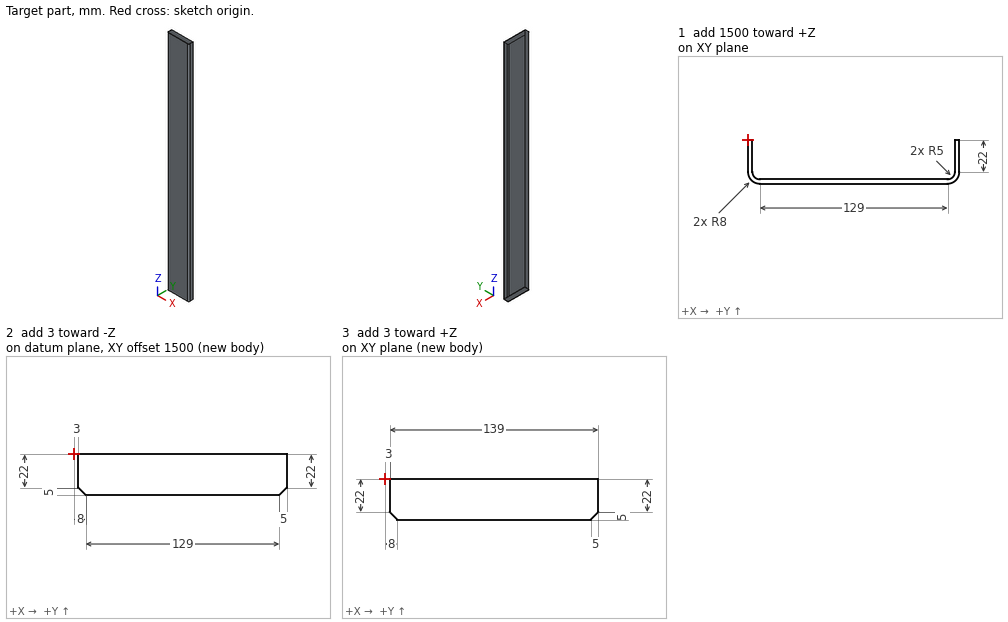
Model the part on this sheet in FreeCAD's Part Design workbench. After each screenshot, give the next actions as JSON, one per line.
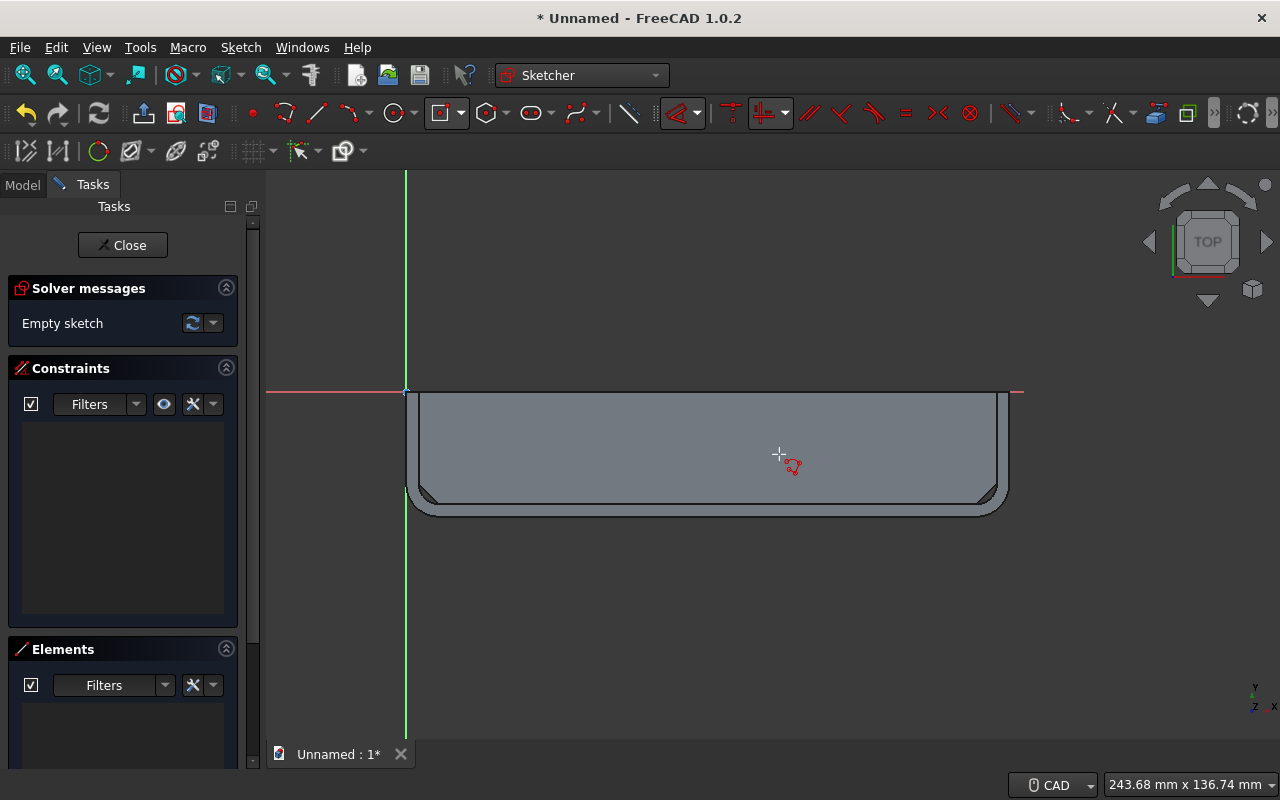
{"action": "scroll", "coordinate": [419, 392], "scroll_direction": "up", "scroll_amount": 2}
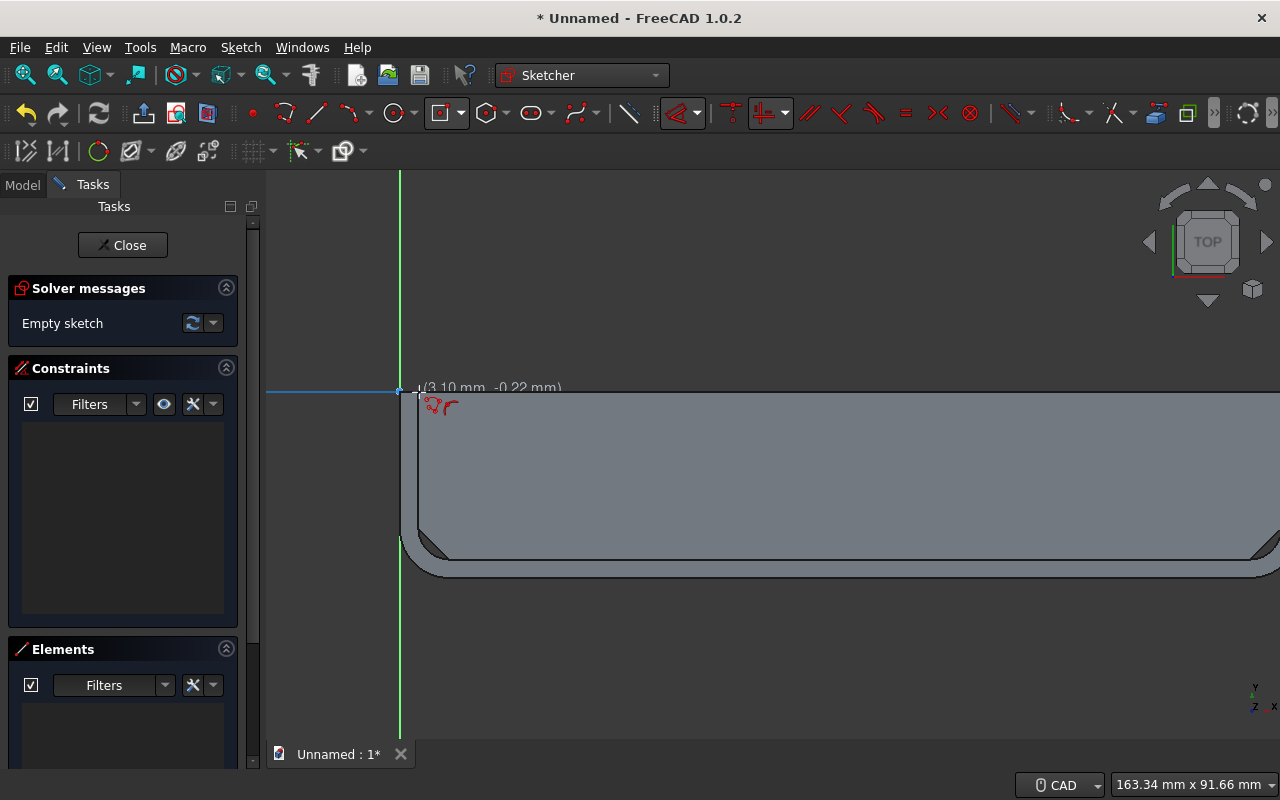
{"action": "left_click", "coordinate": [418, 392]}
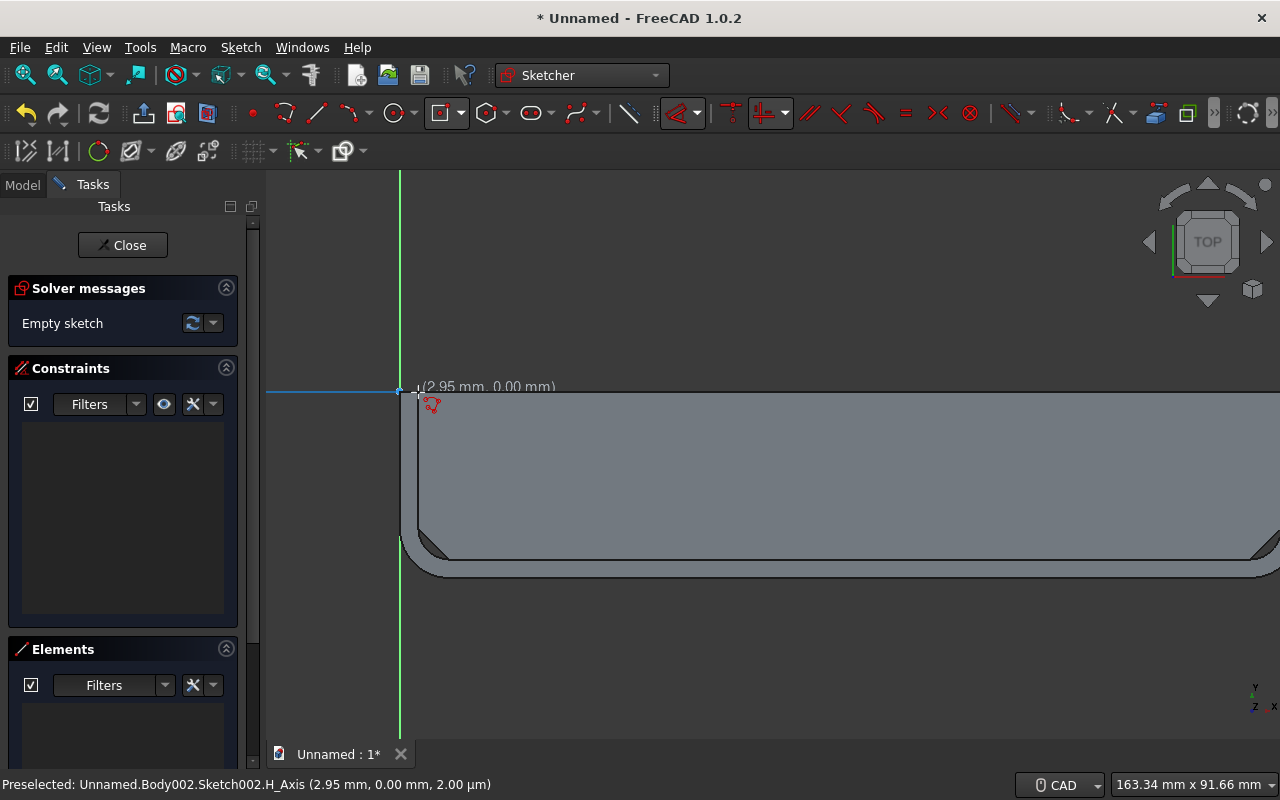
{"action": "scroll", "coordinate": [428, 411], "scroll_direction": "down", "scroll_amount": 2}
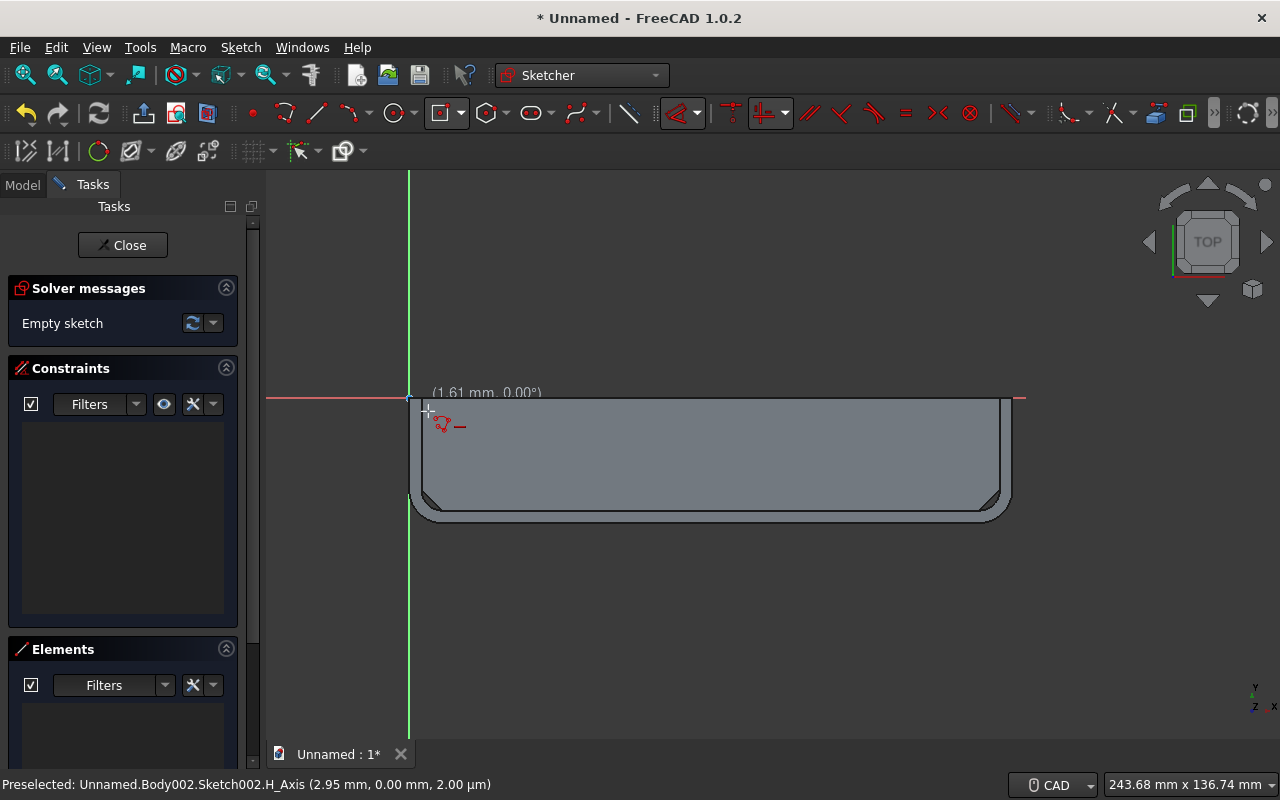
{"action": "left_click", "coordinate": [1000, 407]}
{"action": "left_click", "coordinate": [1000, 490]}
{"action": "left_click", "coordinate": [979, 511]}
{"action": "left_click", "coordinate": [442, 511]}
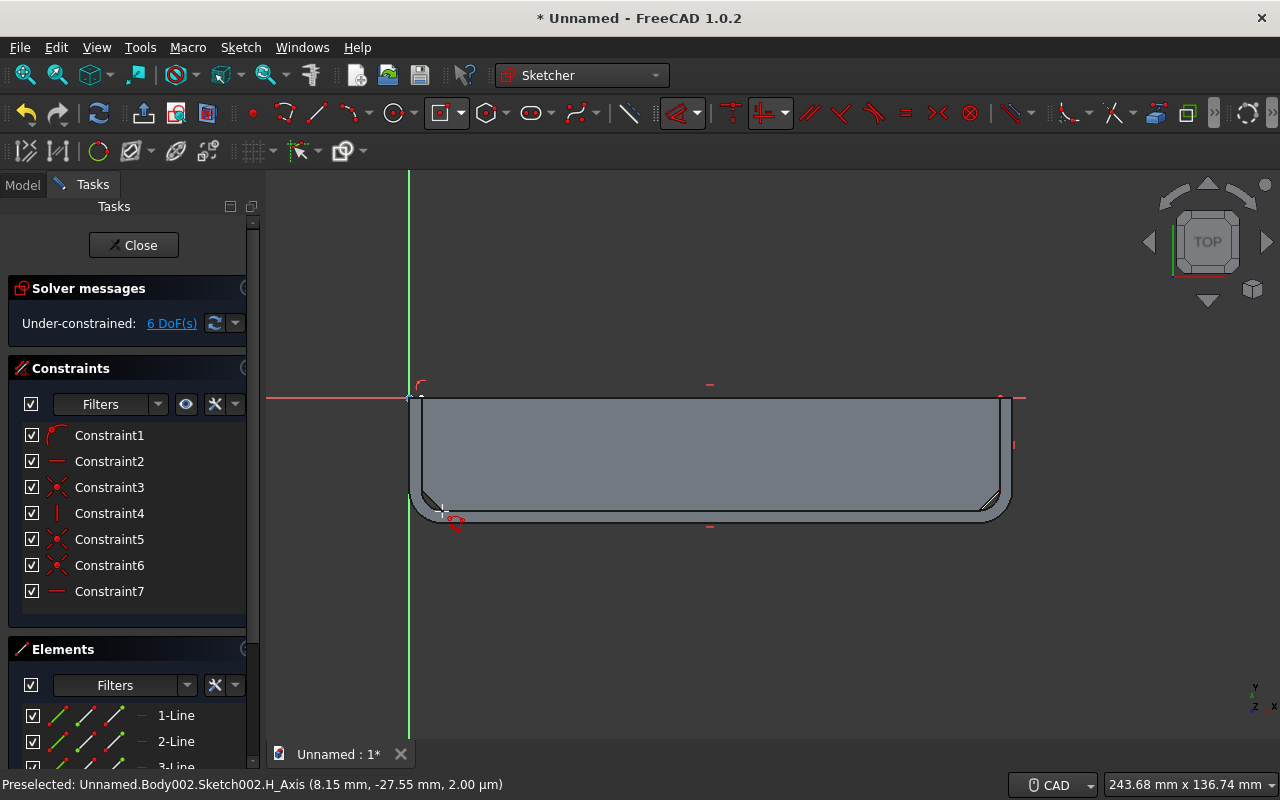
{"action": "scroll", "coordinate": [422, 490], "scroll_direction": "up", "scroll_amount": 2}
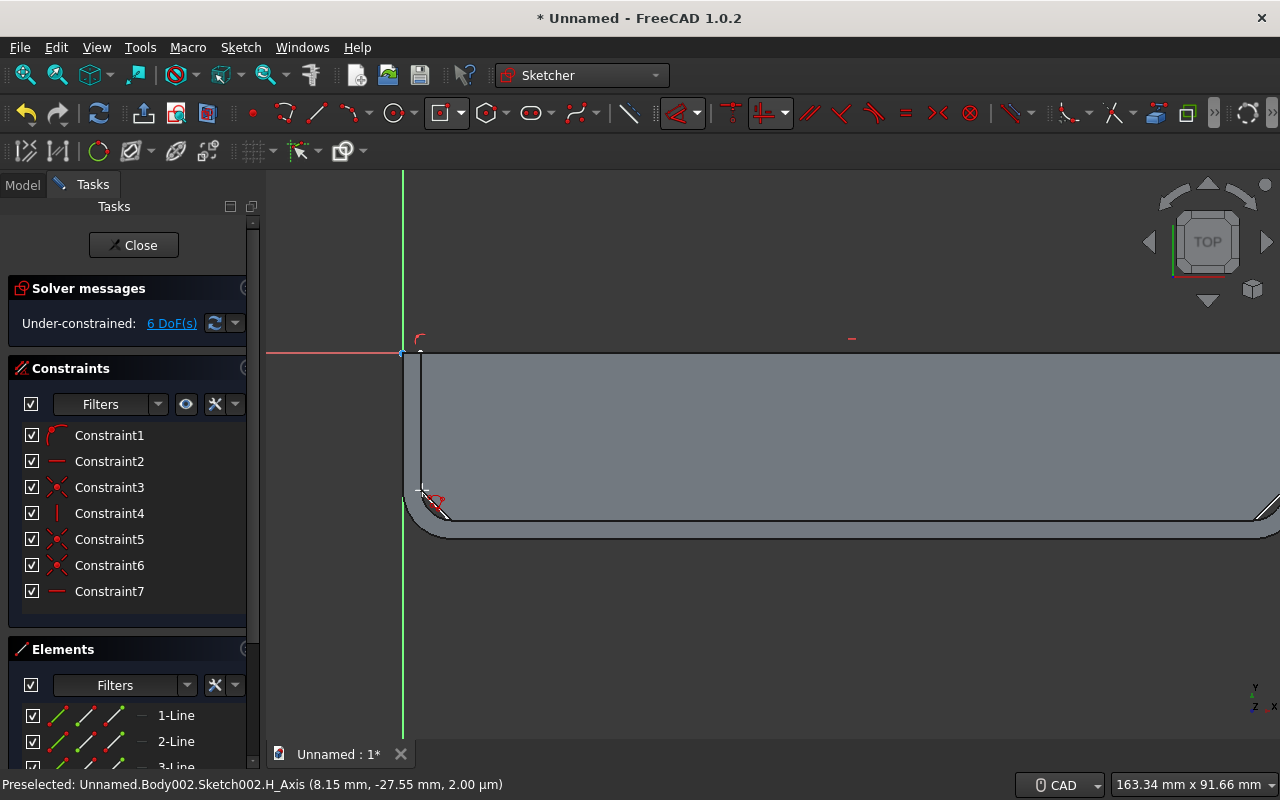
{"action": "left_click", "coordinate": [421, 490]}
{"action": "left_click", "coordinate": [421, 353]}
{"action": "key", "text": "Escape"}
{"action": "key", "text": "Escape"}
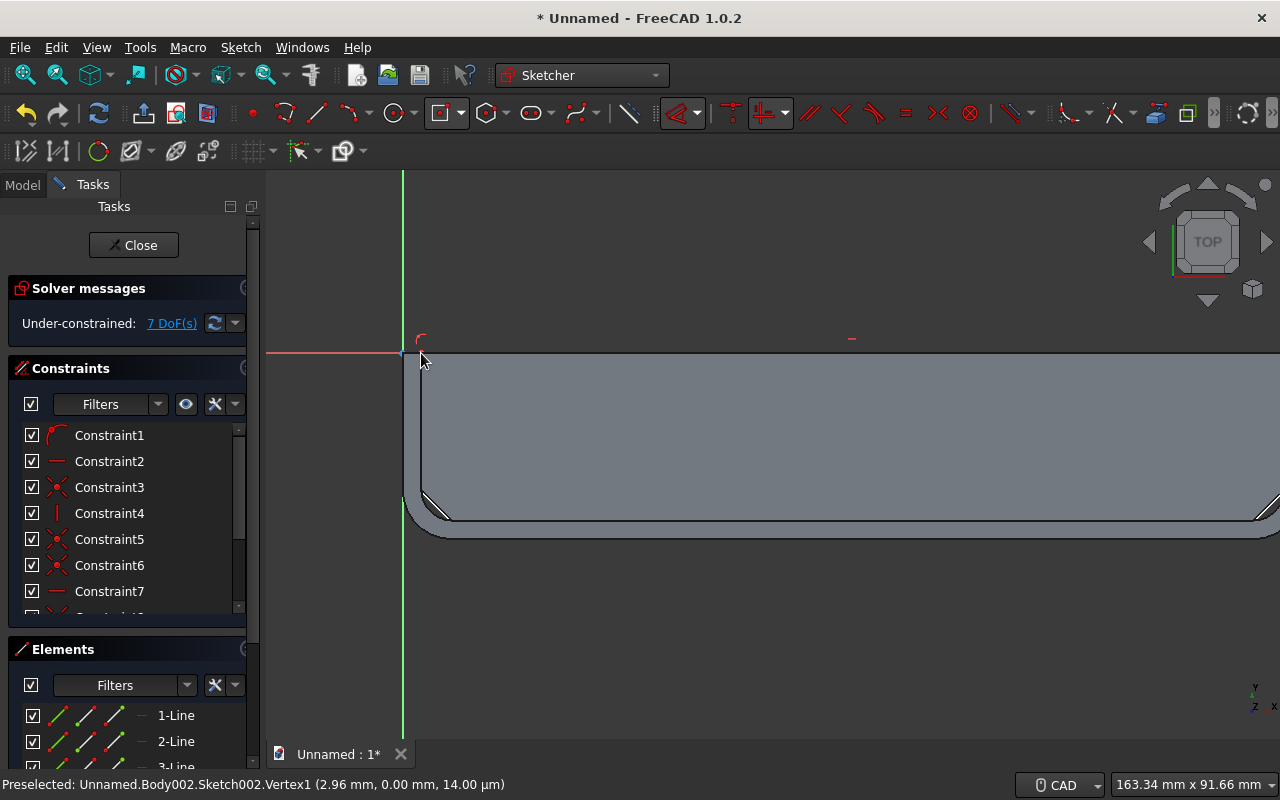
{"action": "scroll", "coordinate": [422, 490], "scroll_direction": "down", "scroll_amount": 2}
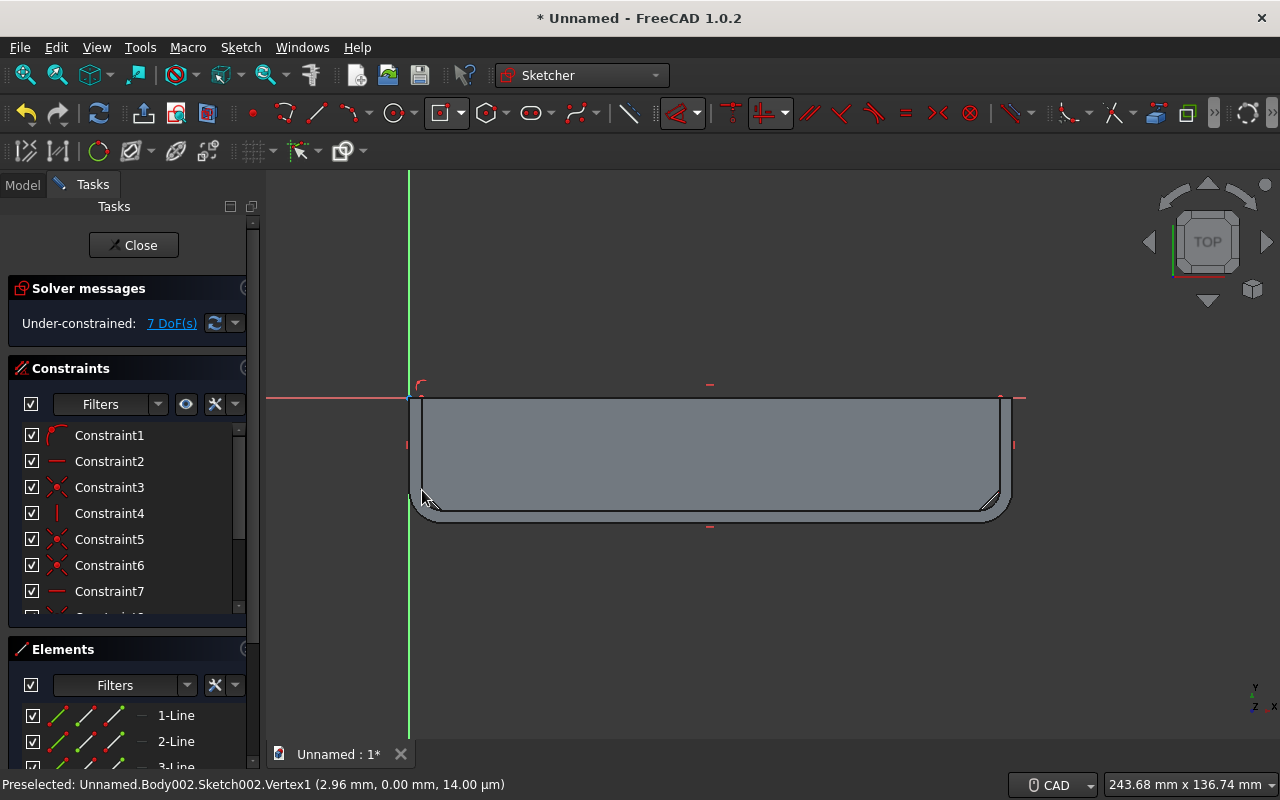
{"action": "left_click", "coordinate": [1000, 426]}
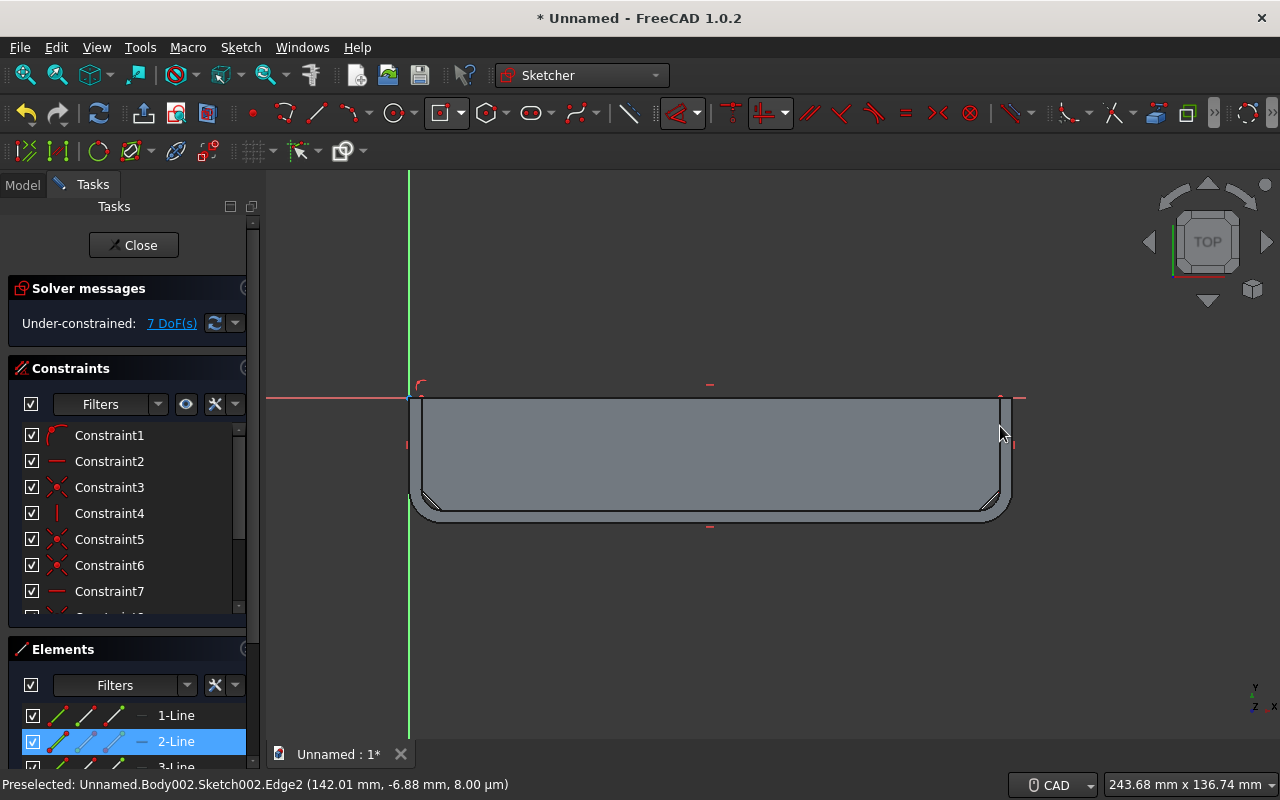
{"action": "key", "text": "i"}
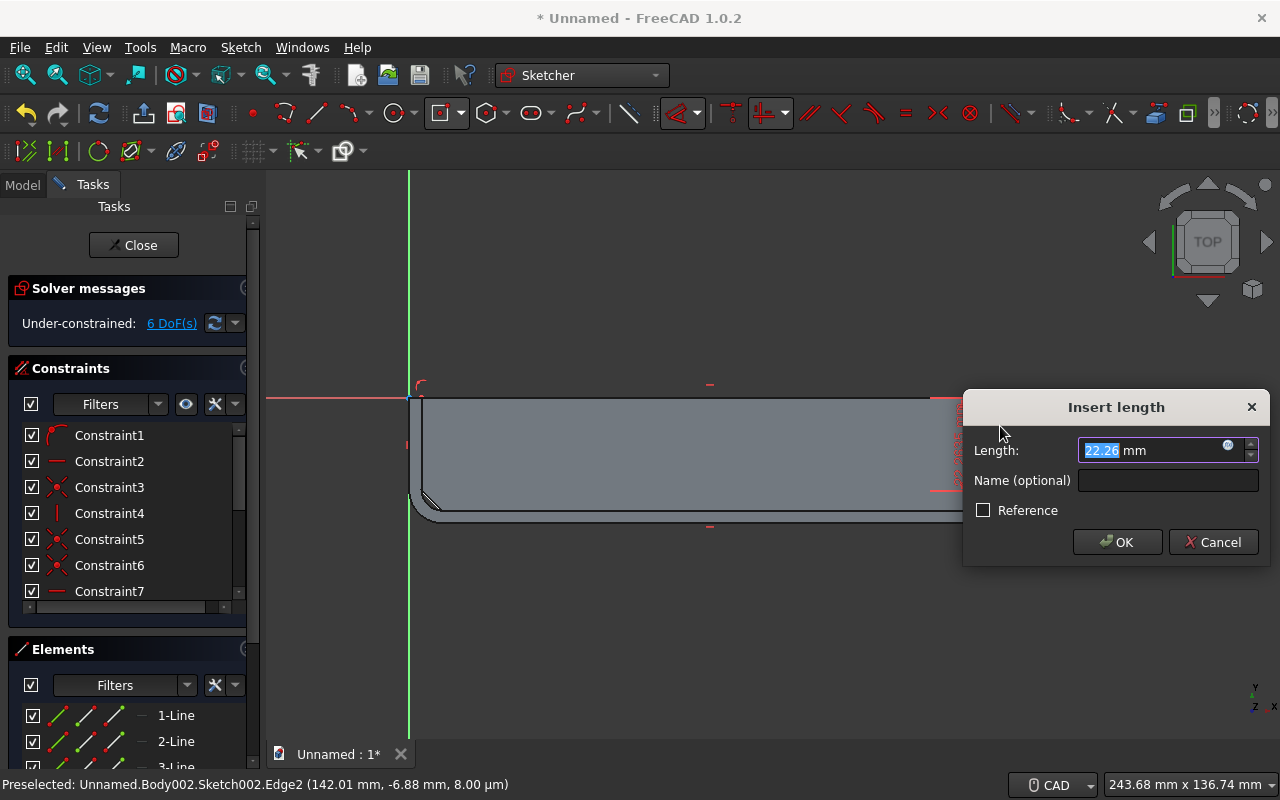
{"action": "type", "text": "22"}
{"action": "key", "text": "Return"}